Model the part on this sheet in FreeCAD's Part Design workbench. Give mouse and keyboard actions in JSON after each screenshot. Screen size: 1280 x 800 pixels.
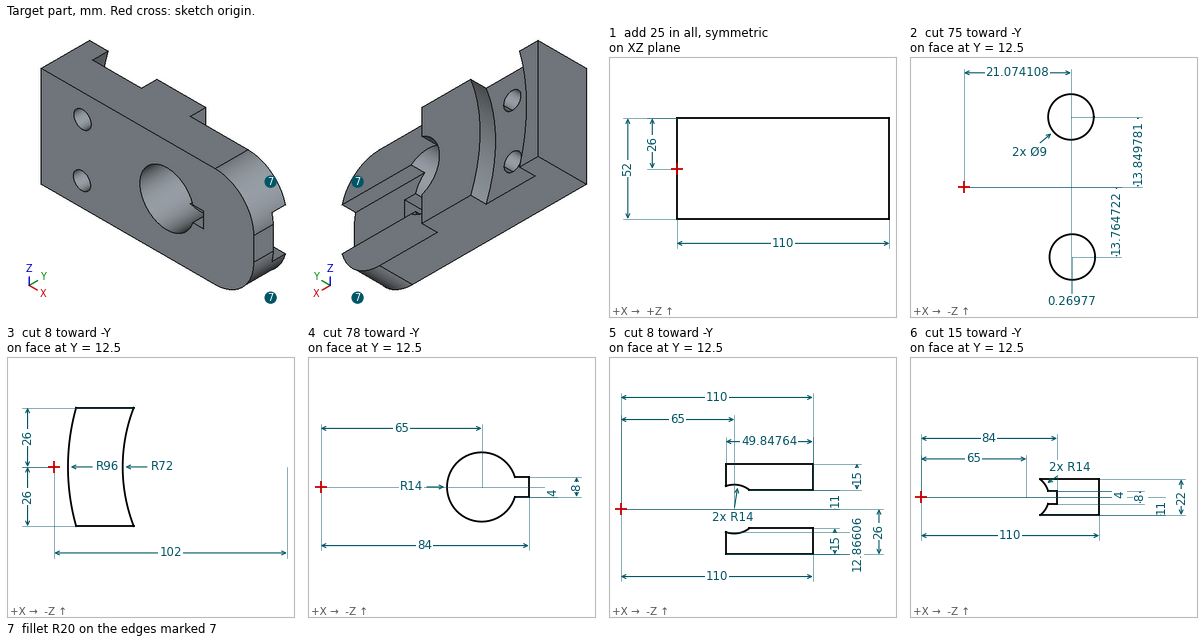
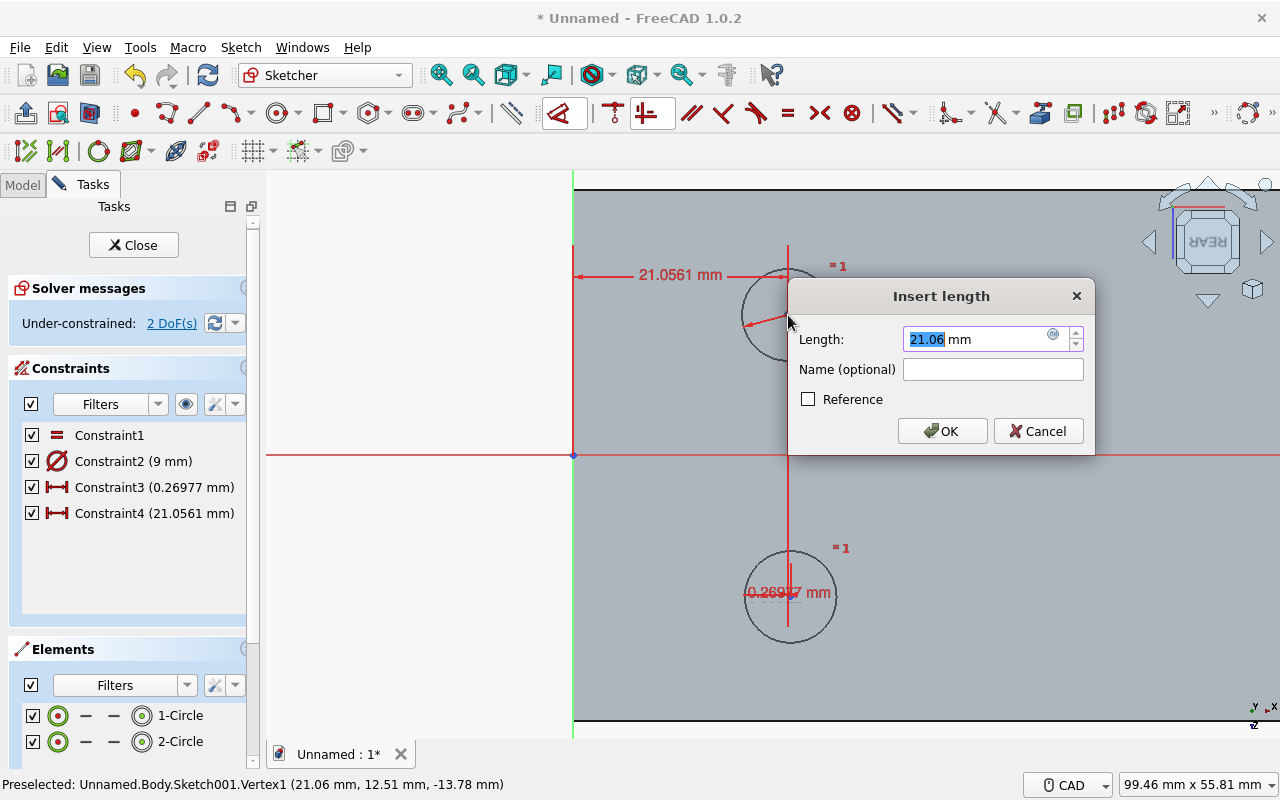
{"action": "type", "text": "21.074108"}
{"action": "key", "text": "Return"}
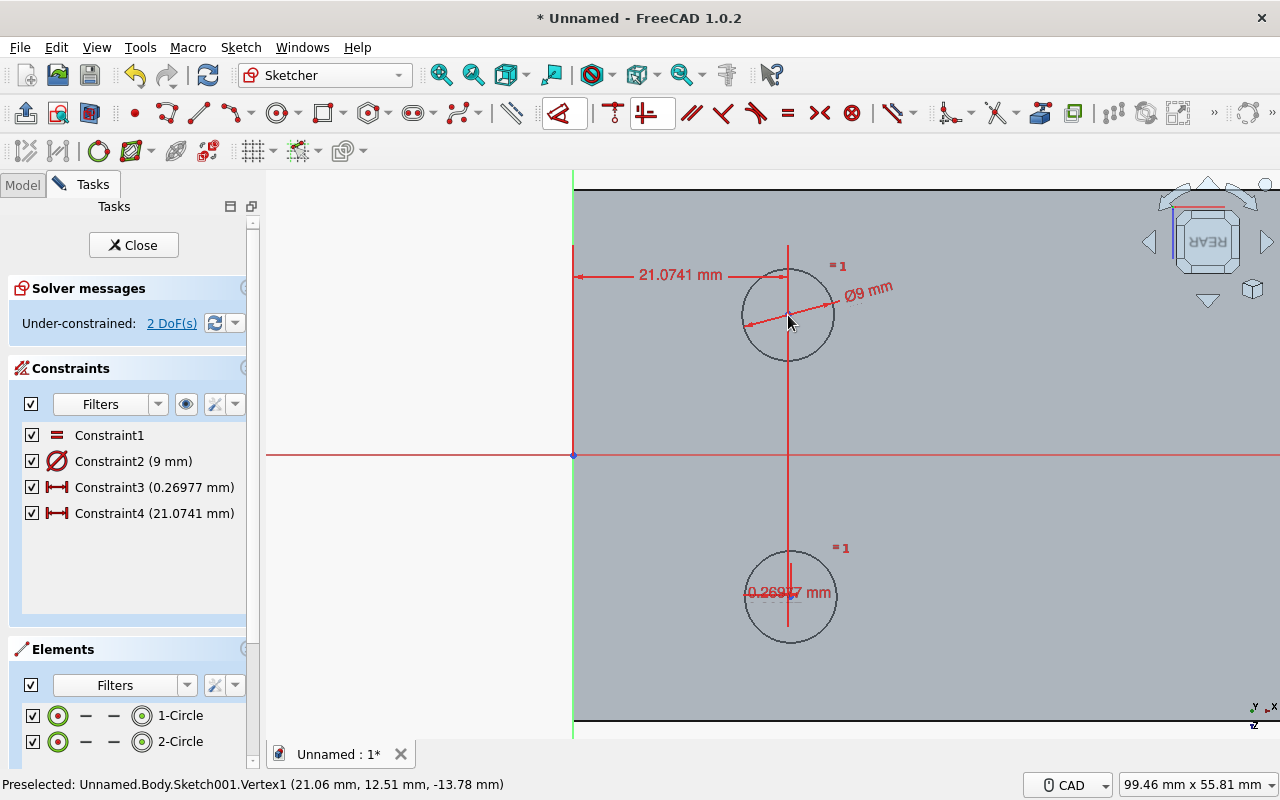
{"action": "left_click", "coordinate": [788, 315]}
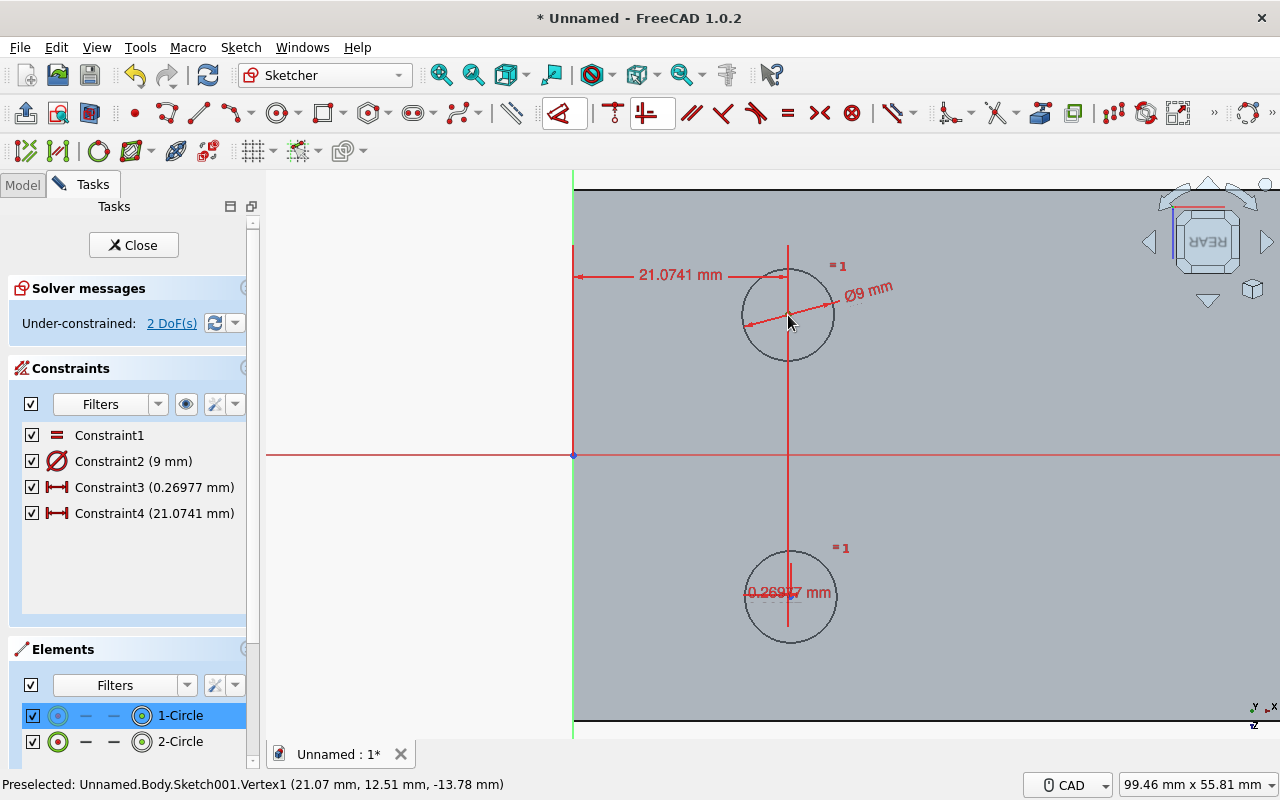
{"action": "left_click", "coordinate": [582, 114]}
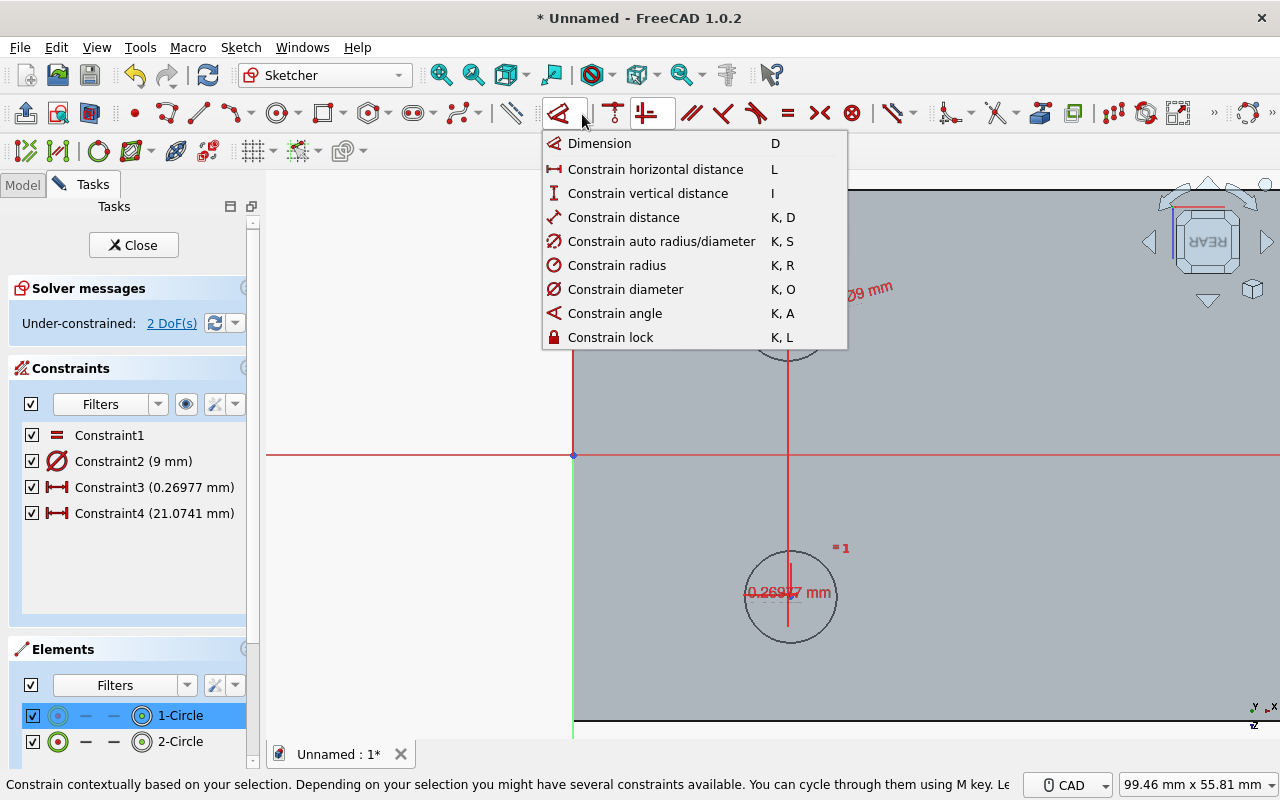
{"action": "left_click", "coordinate": [695, 193]}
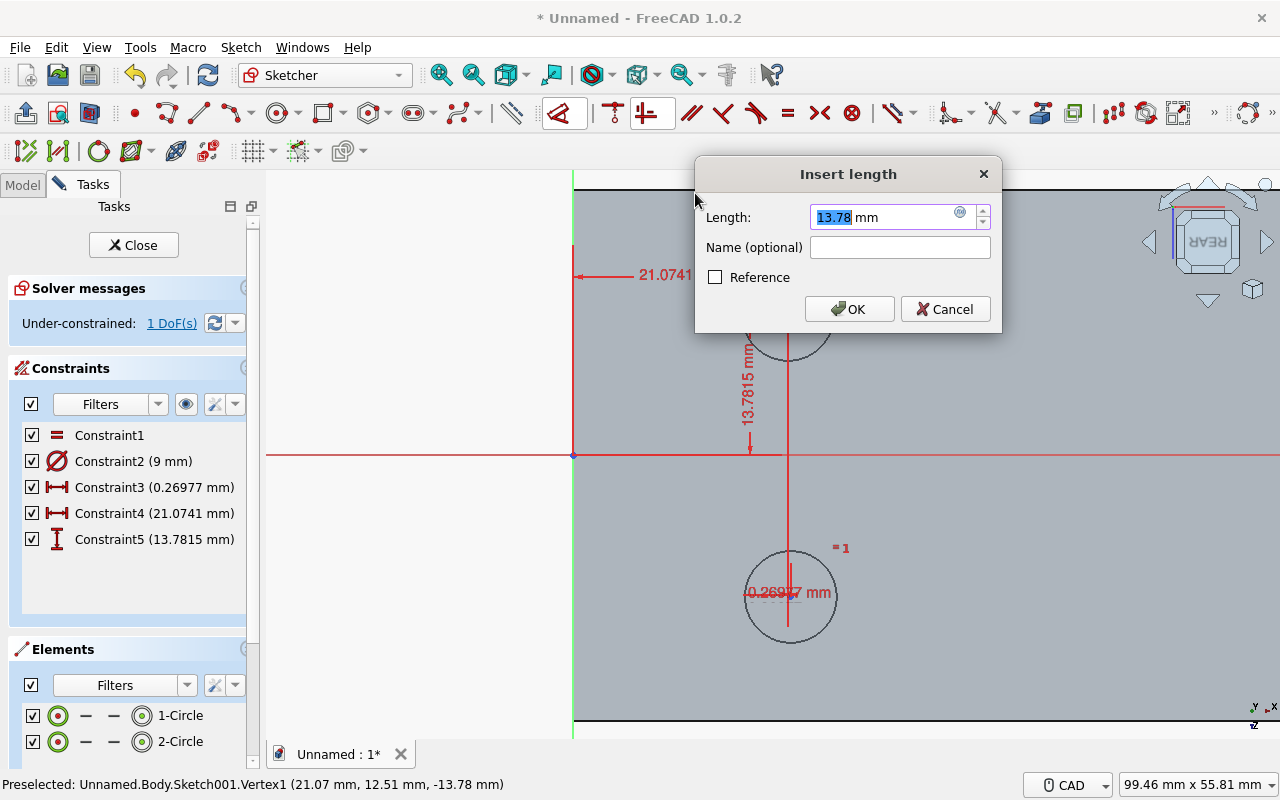
{"action": "type", "text": "13.849781"}
{"action": "key", "text": "Return"}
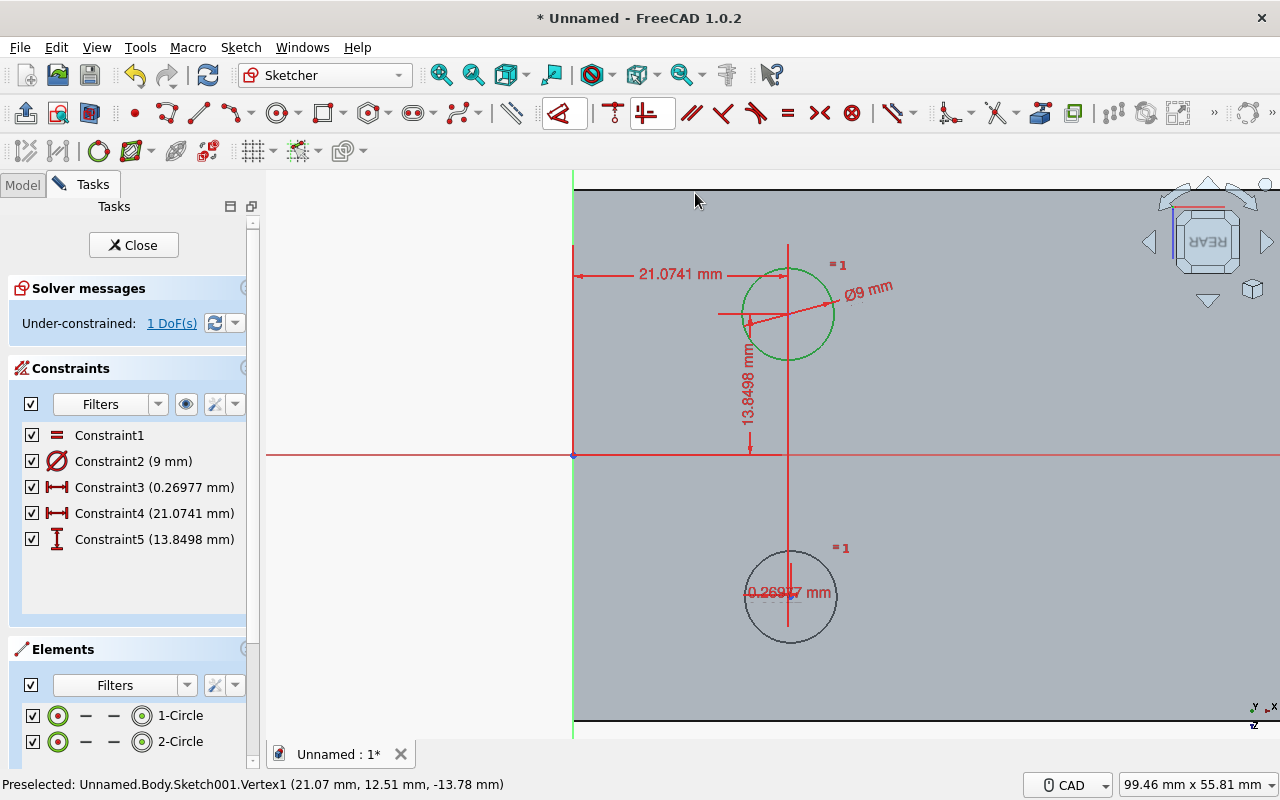
{"action": "left_click", "coordinate": [791, 597]}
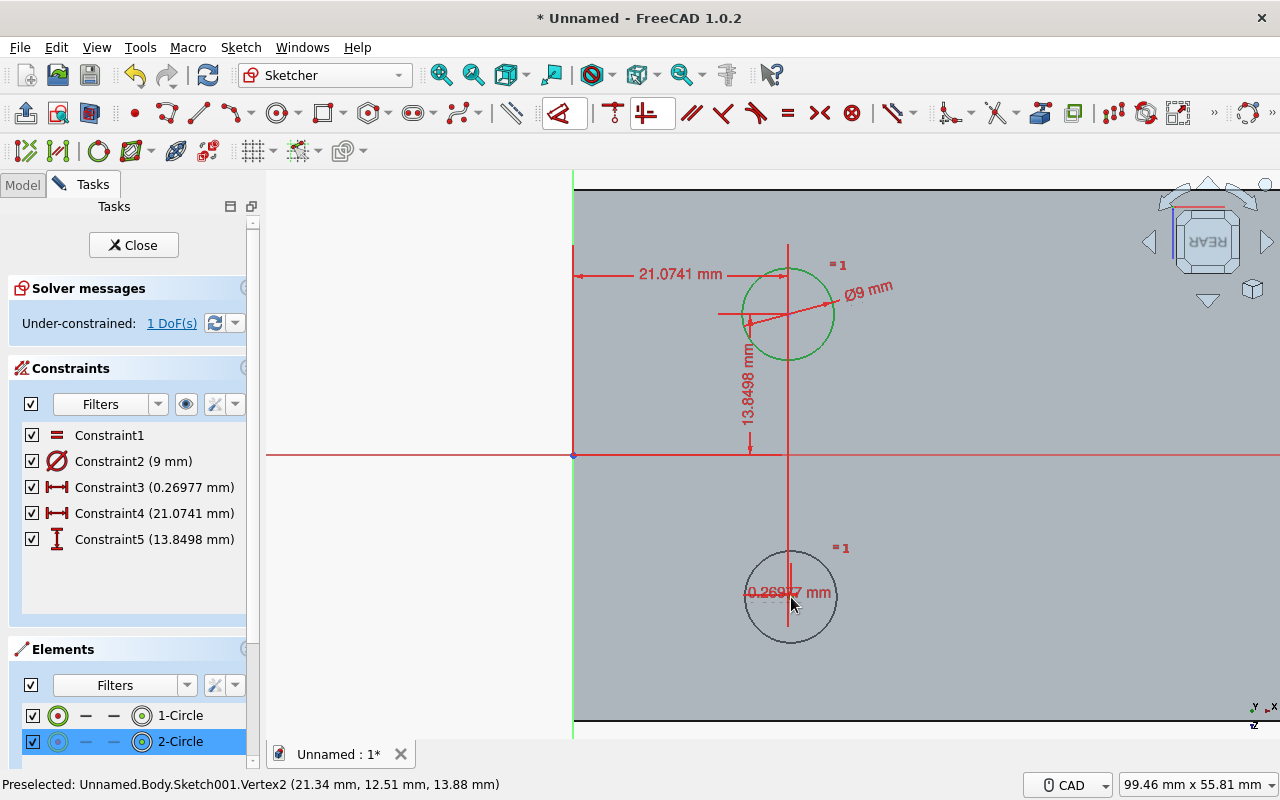
{"action": "left_click", "coordinate": [582, 114]}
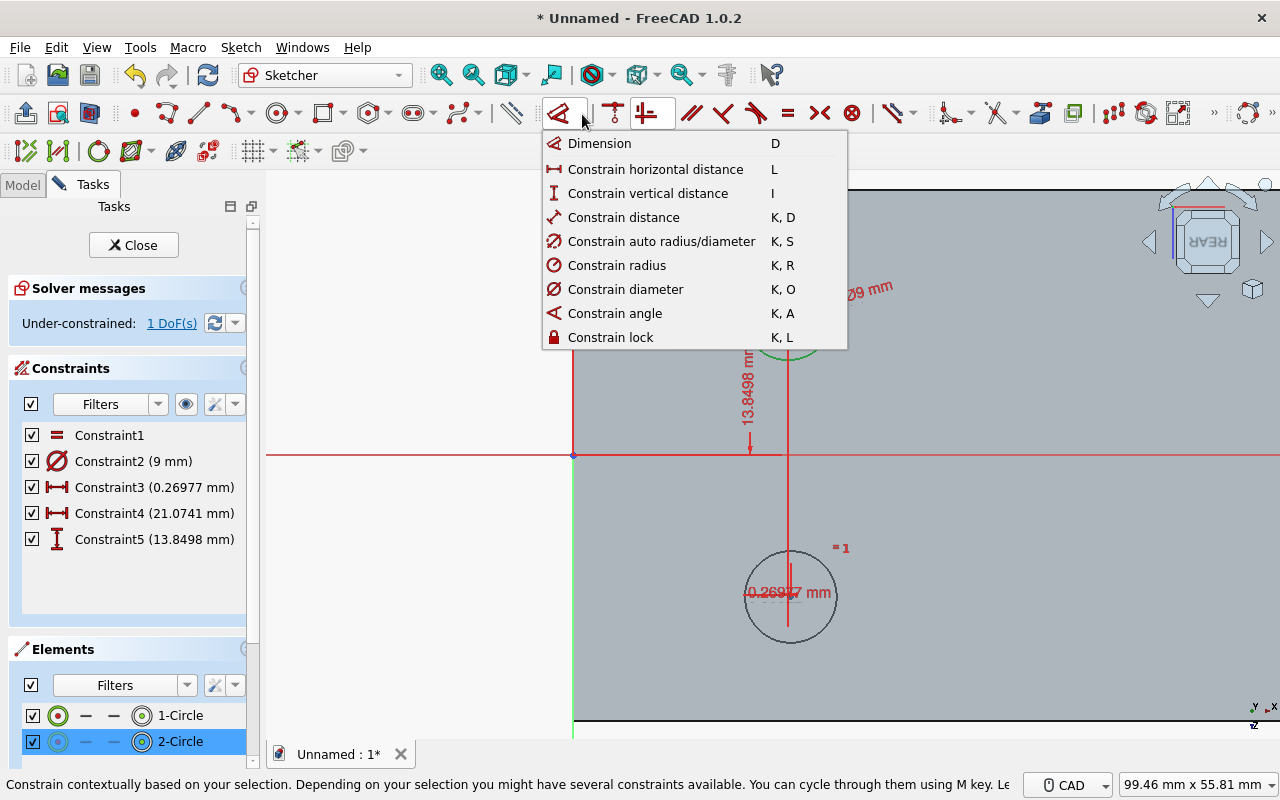
{"action": "left_click", "coordinate": [695, 193]}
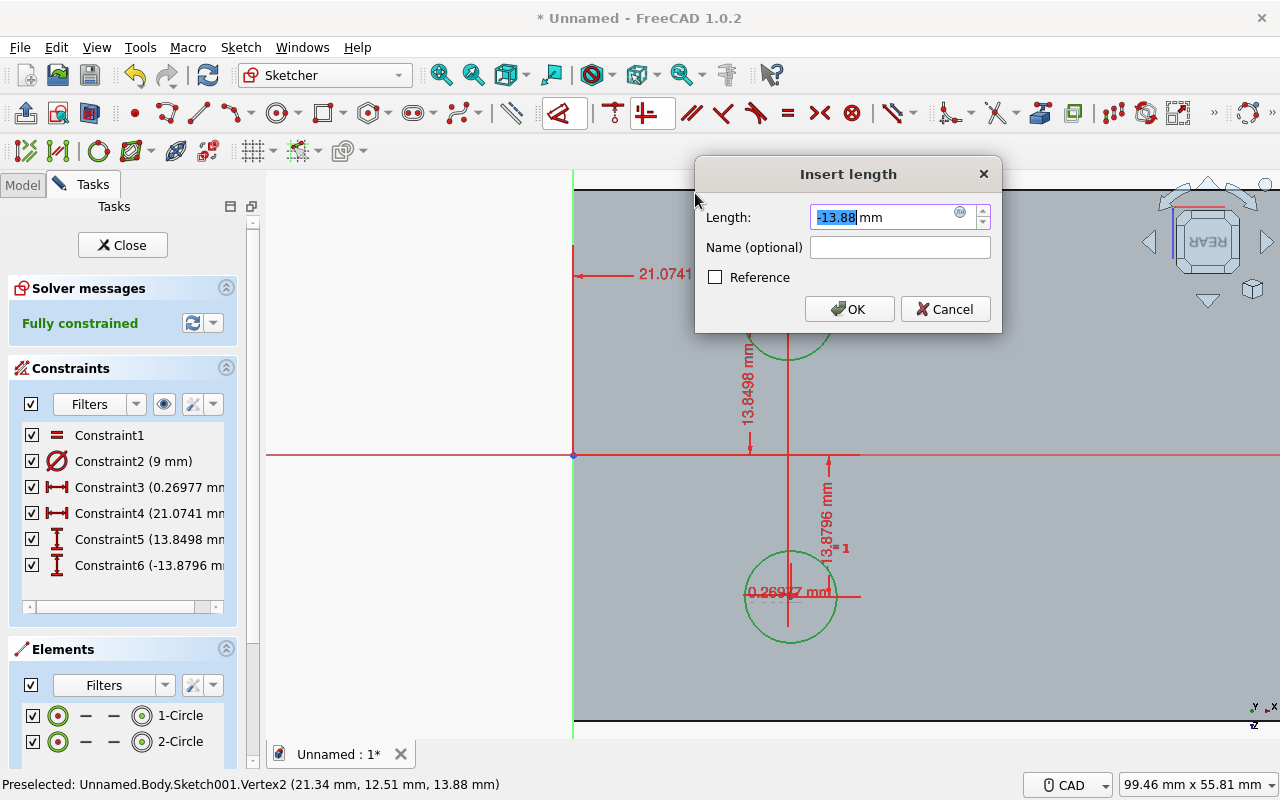
{"action": "type", "text": "-13.764722"}
{"action": "key", "text": "Return"}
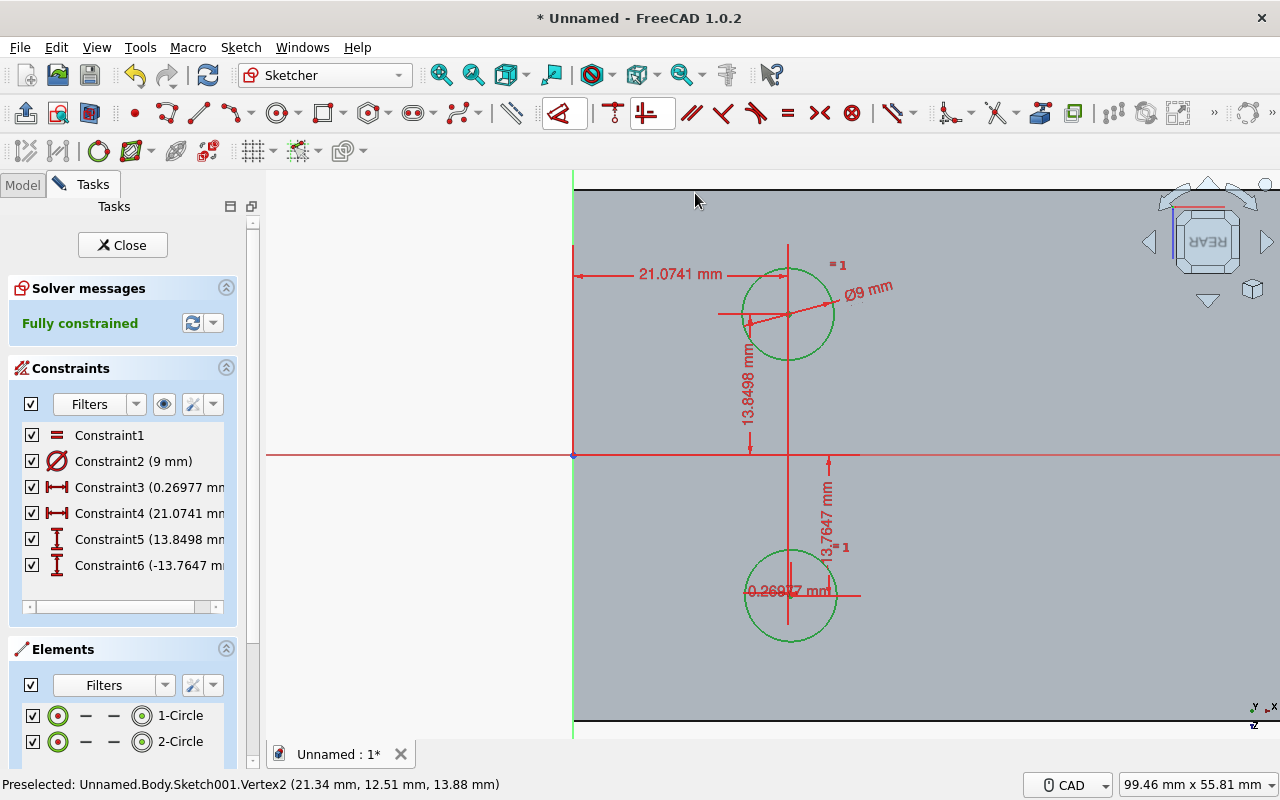
{"action": "left_click", "coordinate": [123, 245]}